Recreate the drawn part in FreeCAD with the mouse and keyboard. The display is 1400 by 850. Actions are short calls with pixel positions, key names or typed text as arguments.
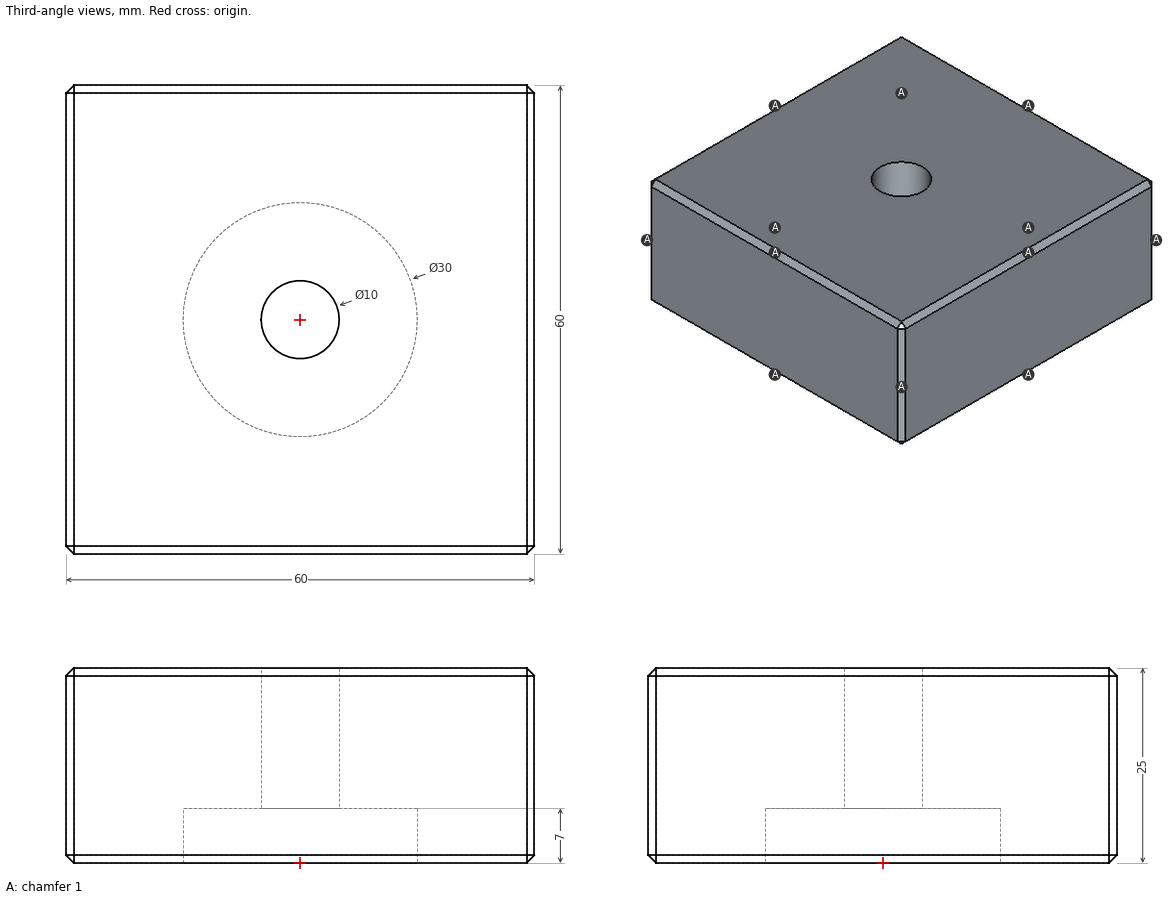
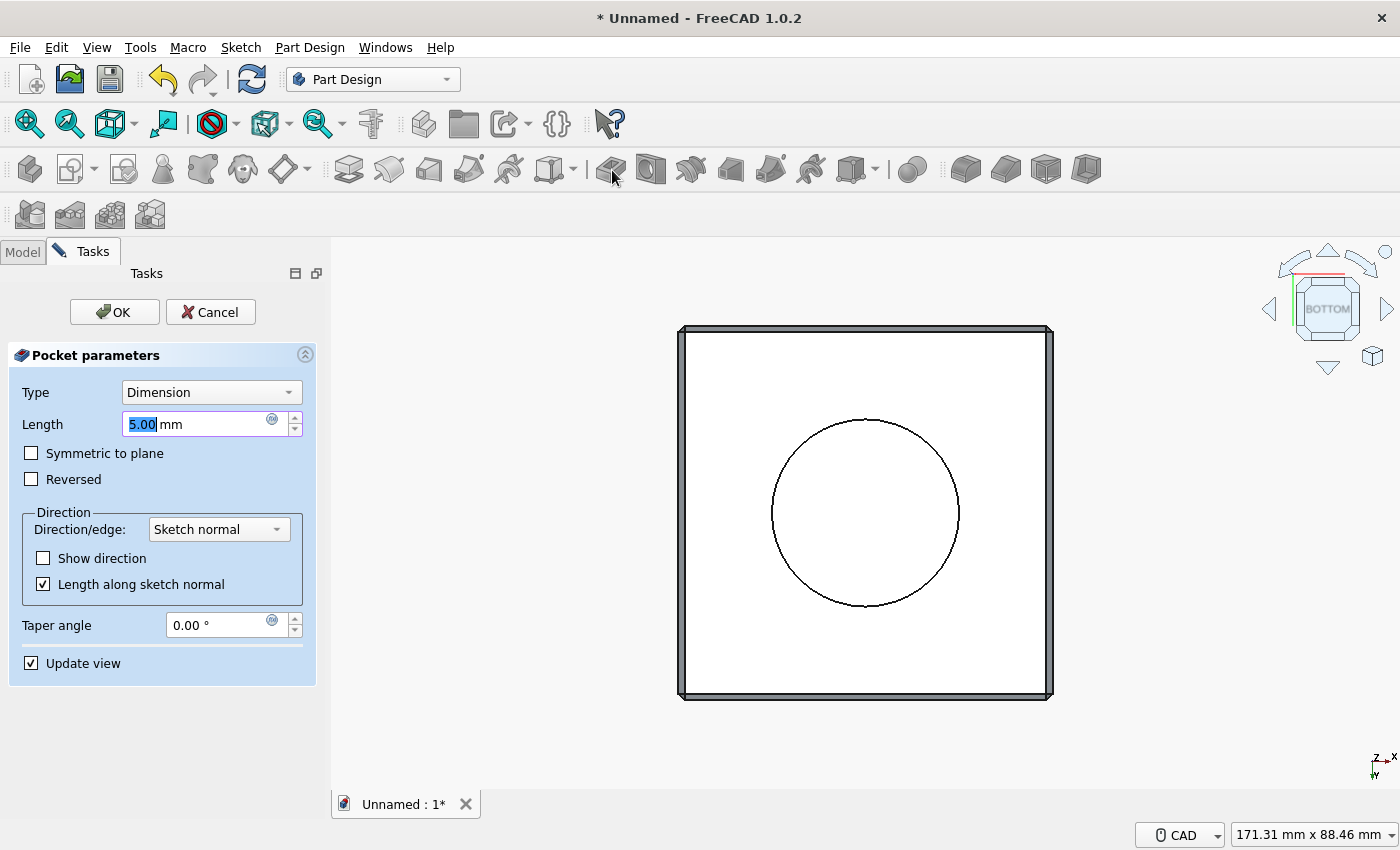
text(7)
key(Tab)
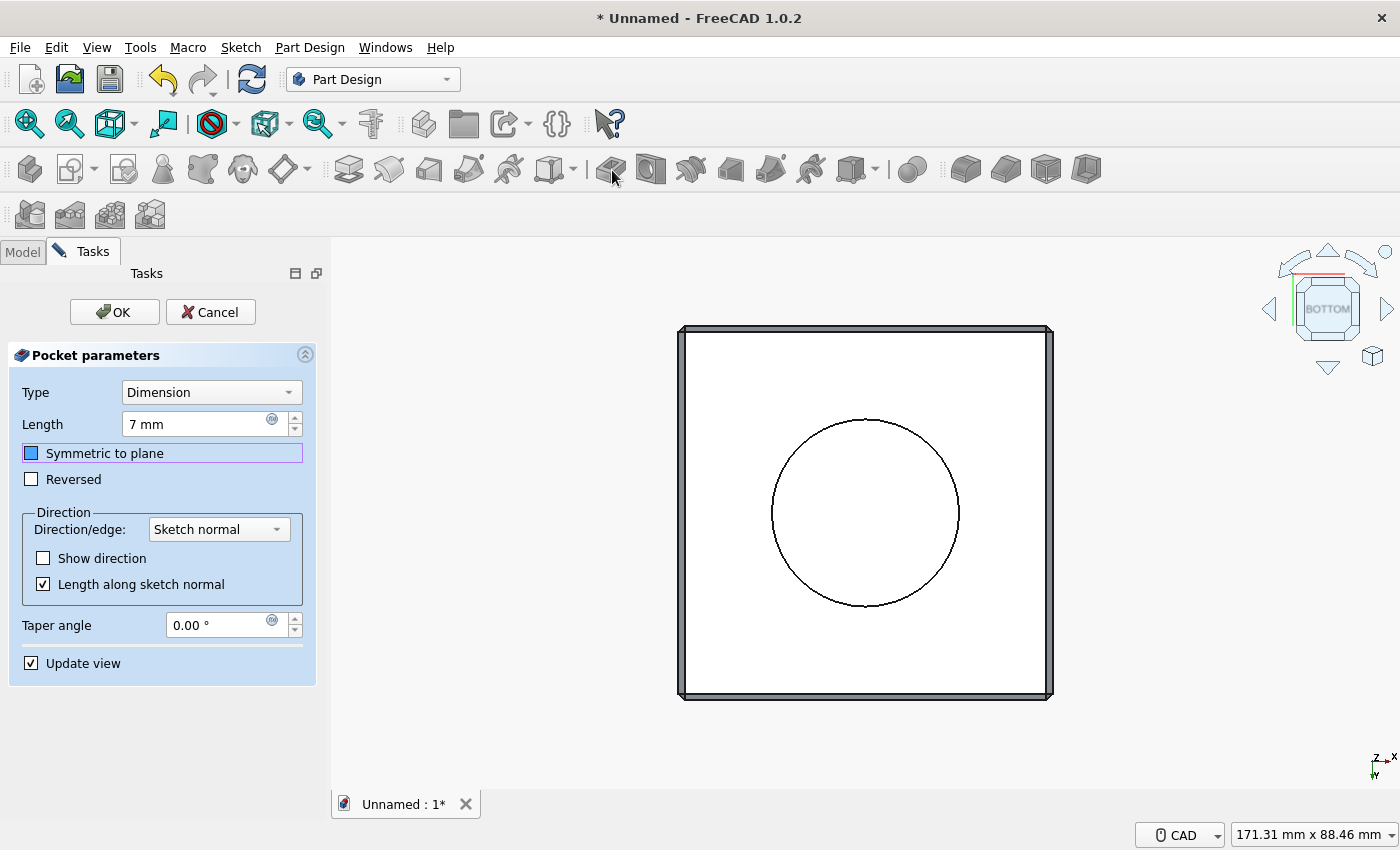
click(115, 312)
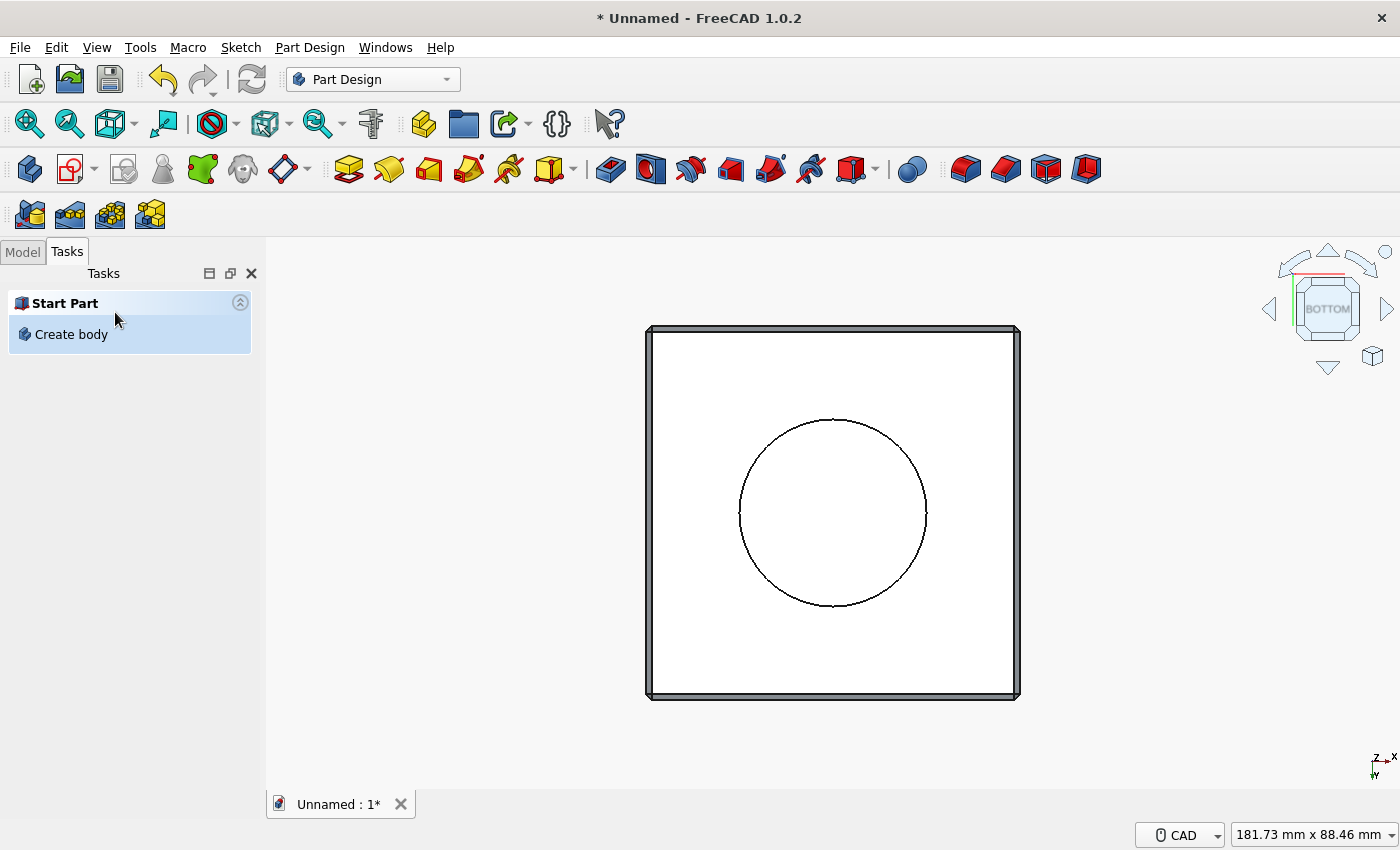
click(833, 512)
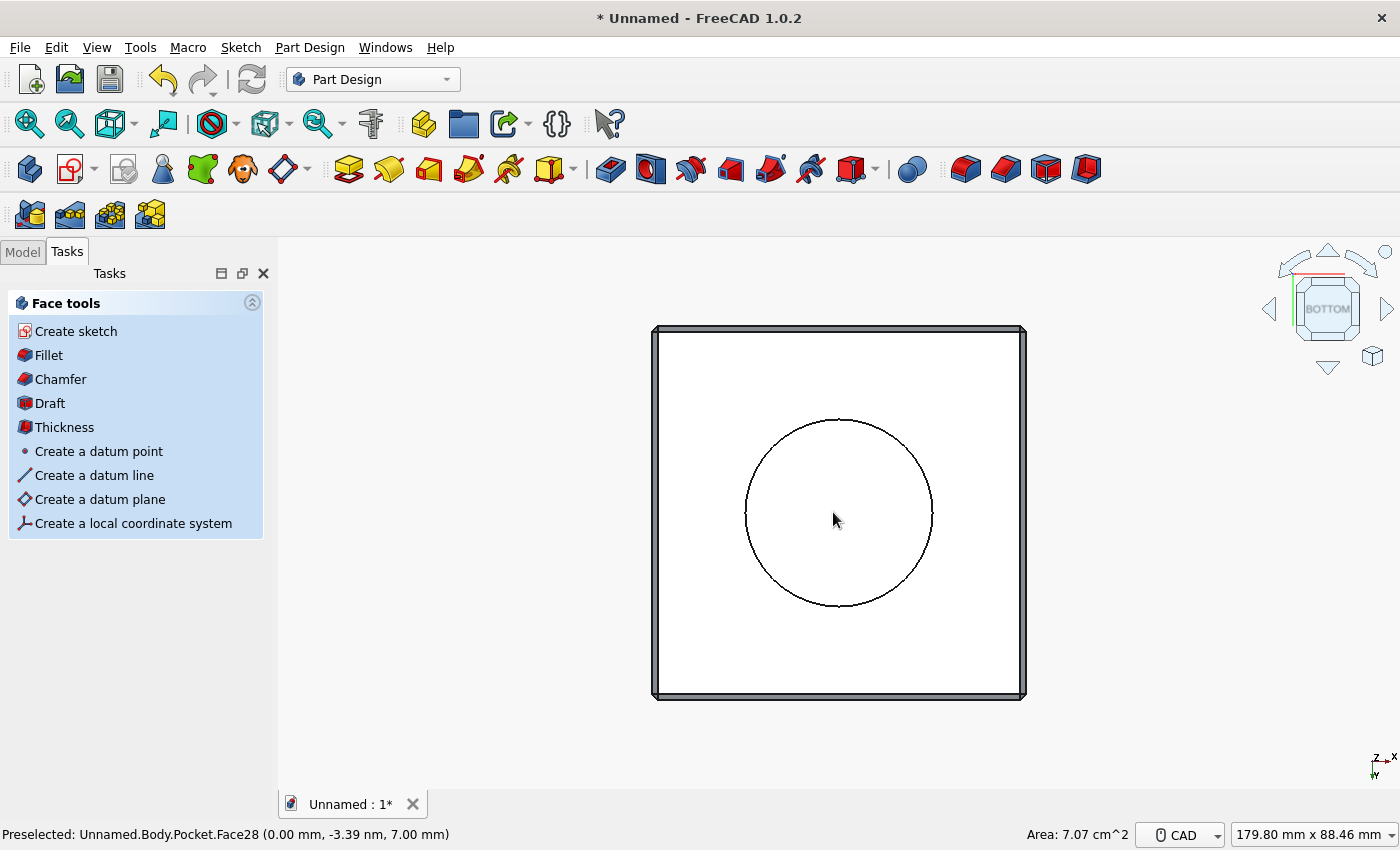
click(70, 170)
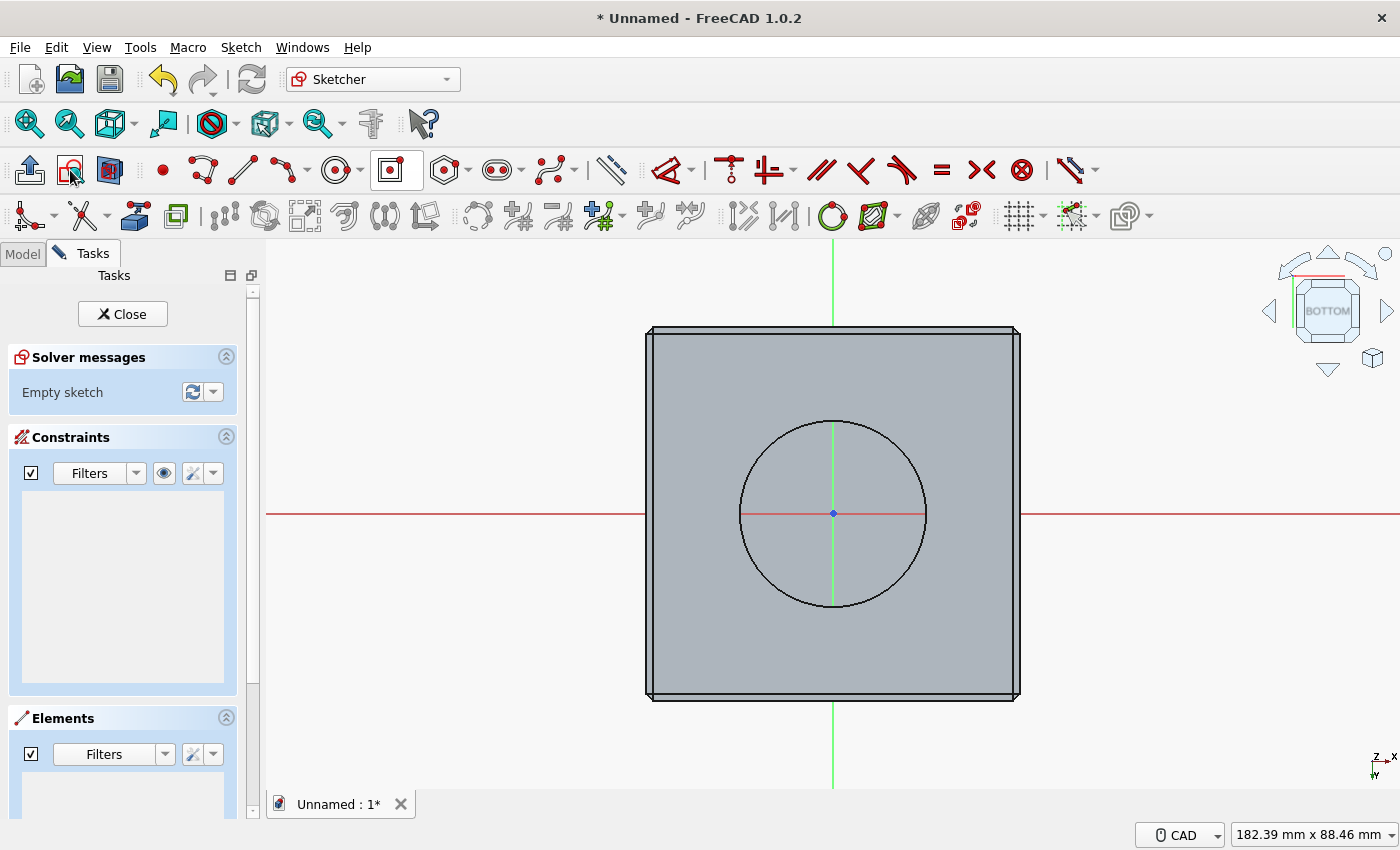
scroll(847, 514, up, 9)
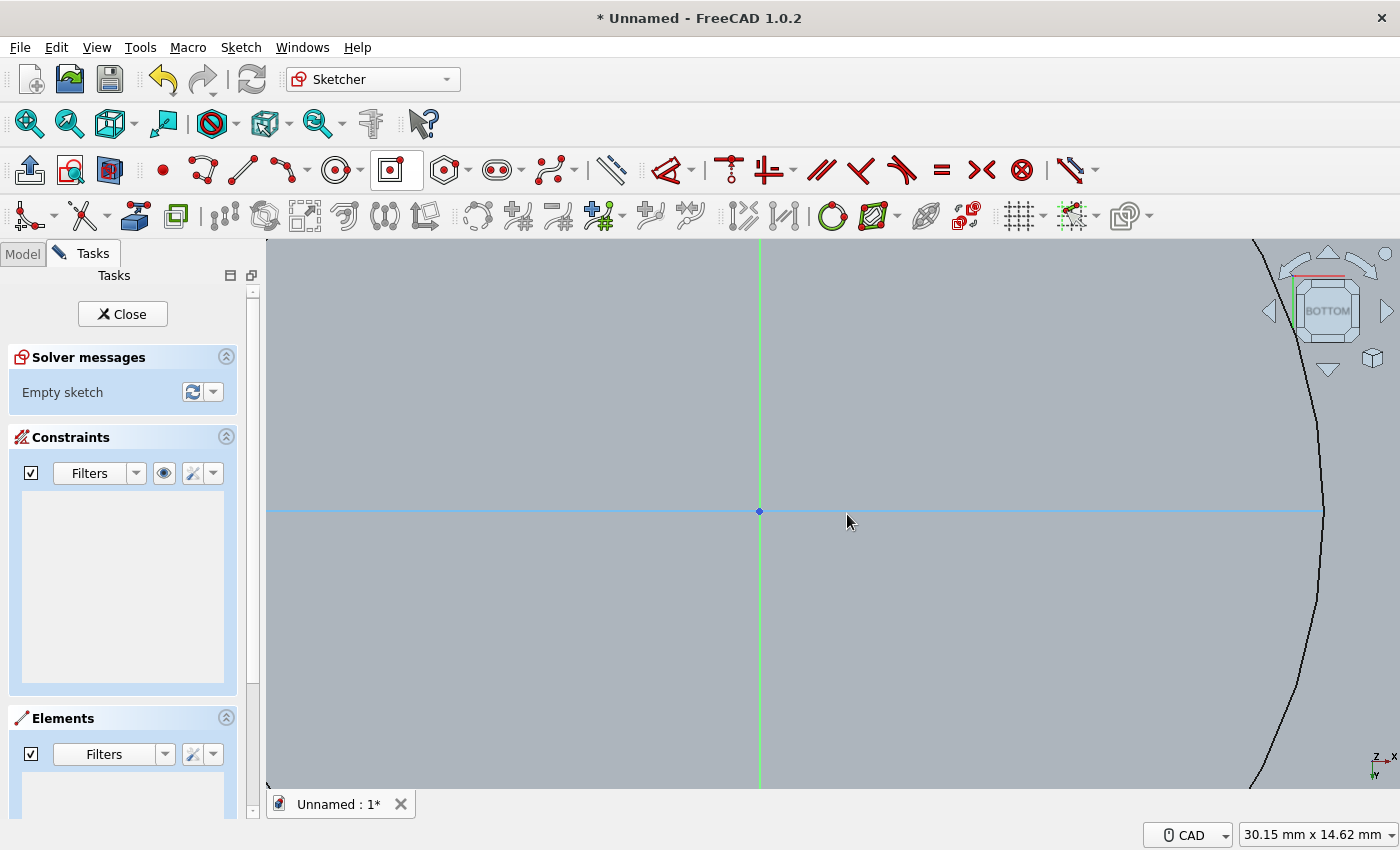
click(336, 170)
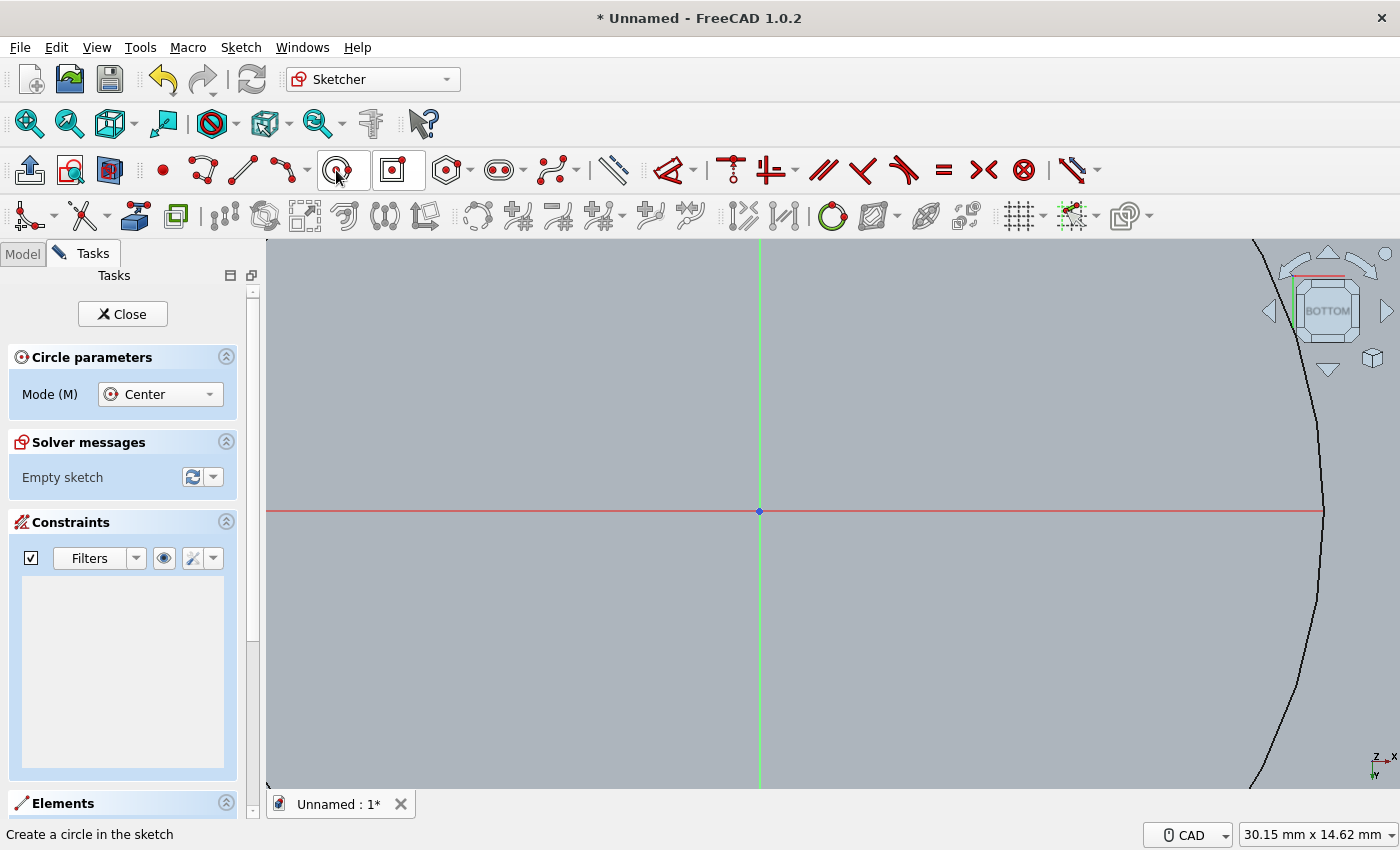
click(760, 511)
move(893, 378)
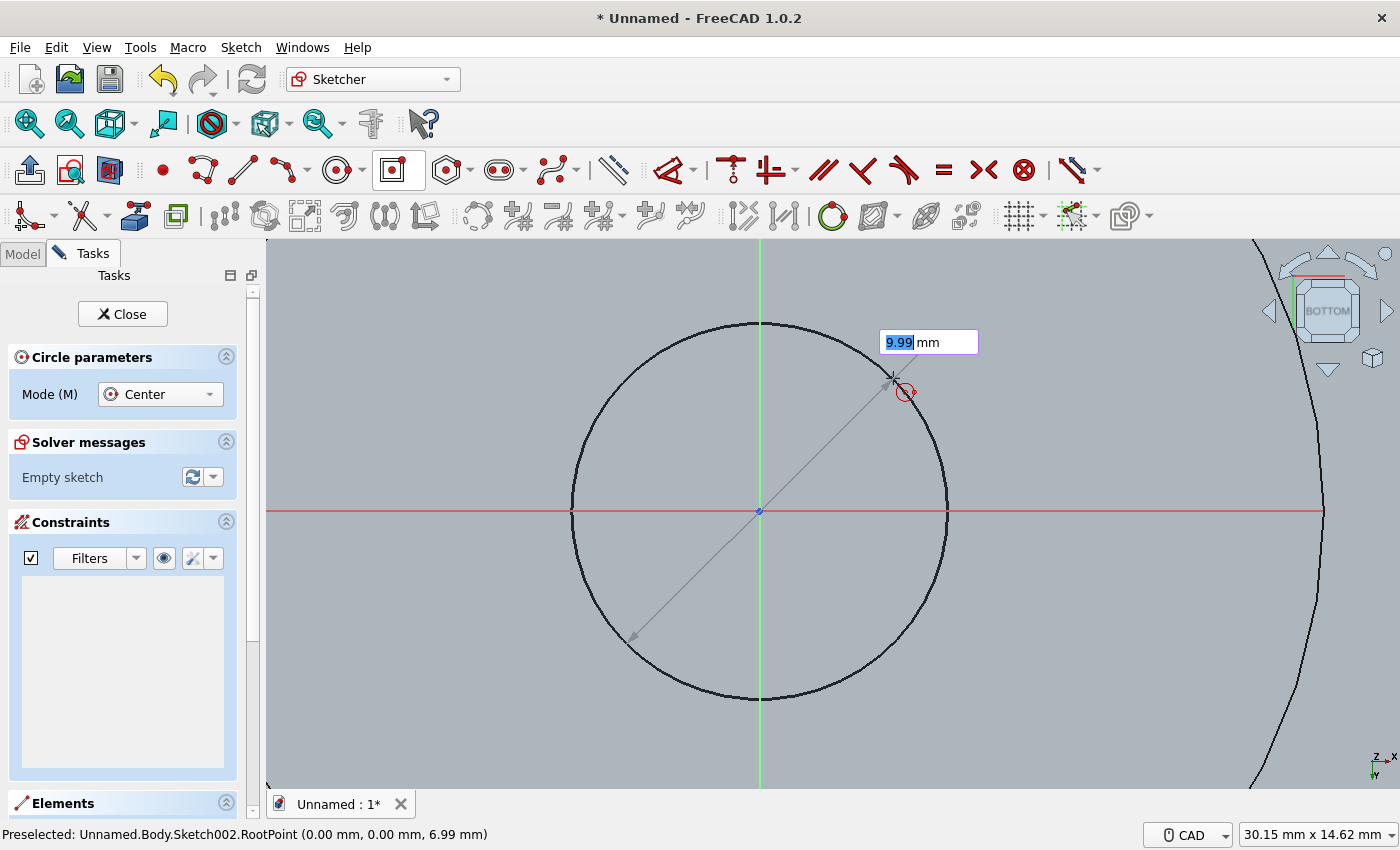
text(10)
key(Return)
key(Escape)